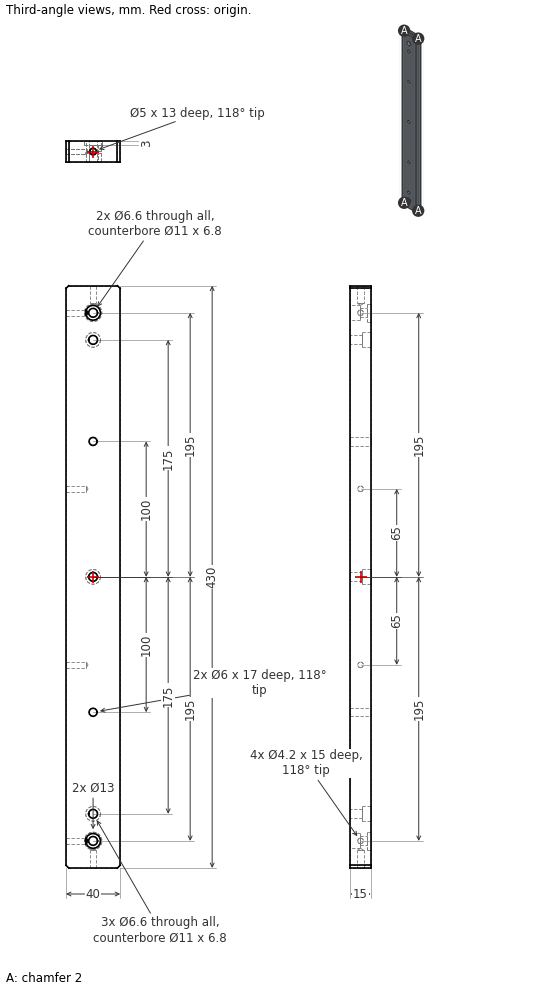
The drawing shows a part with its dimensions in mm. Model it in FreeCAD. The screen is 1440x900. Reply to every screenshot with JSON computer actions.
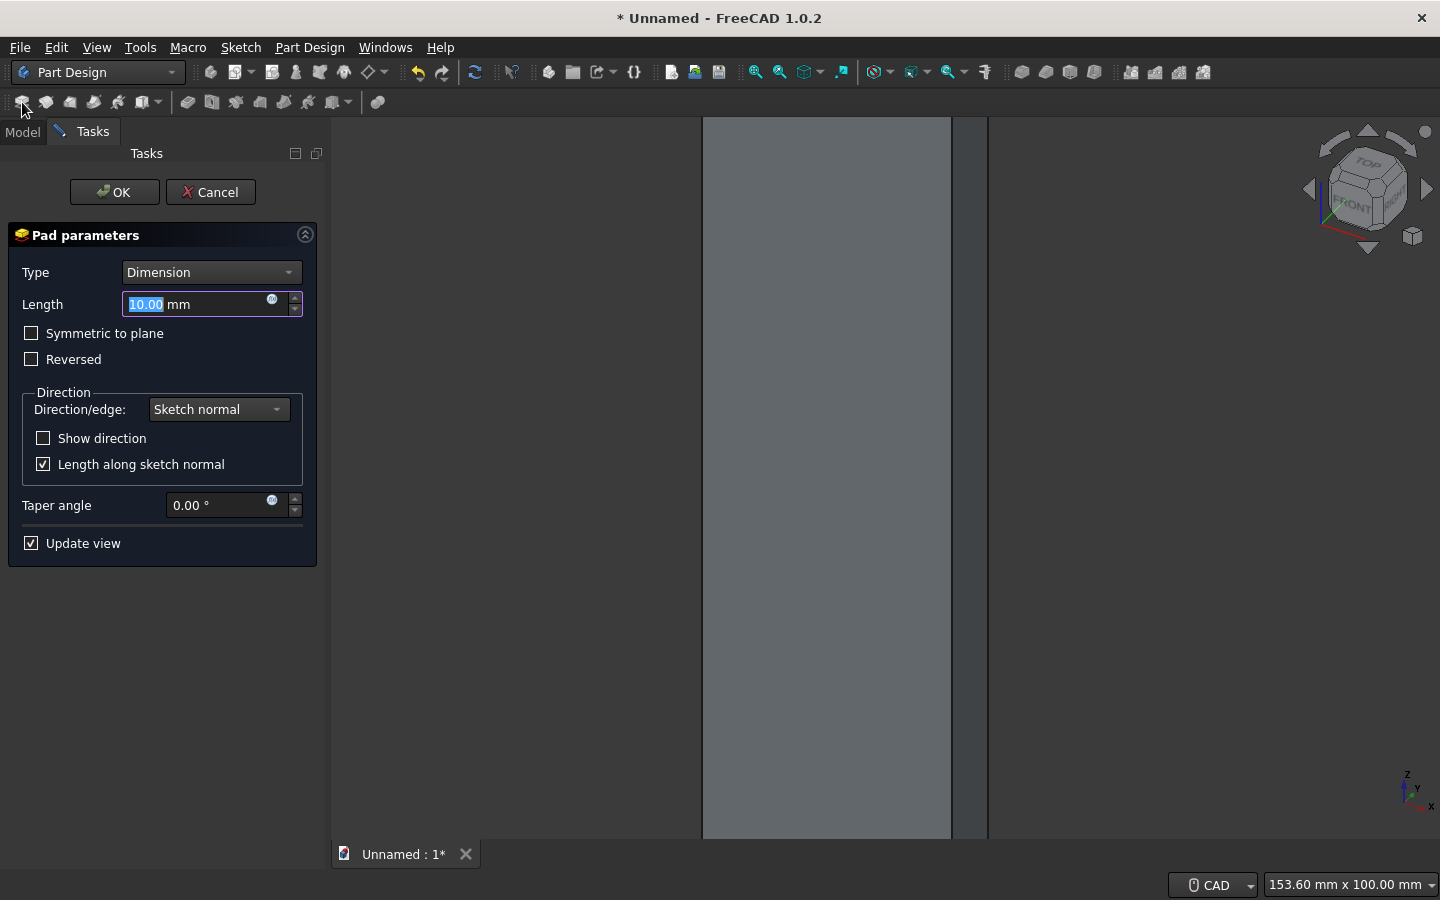
{"action": "type", "text": "15"}
{"action": "key", "text": "Tab"}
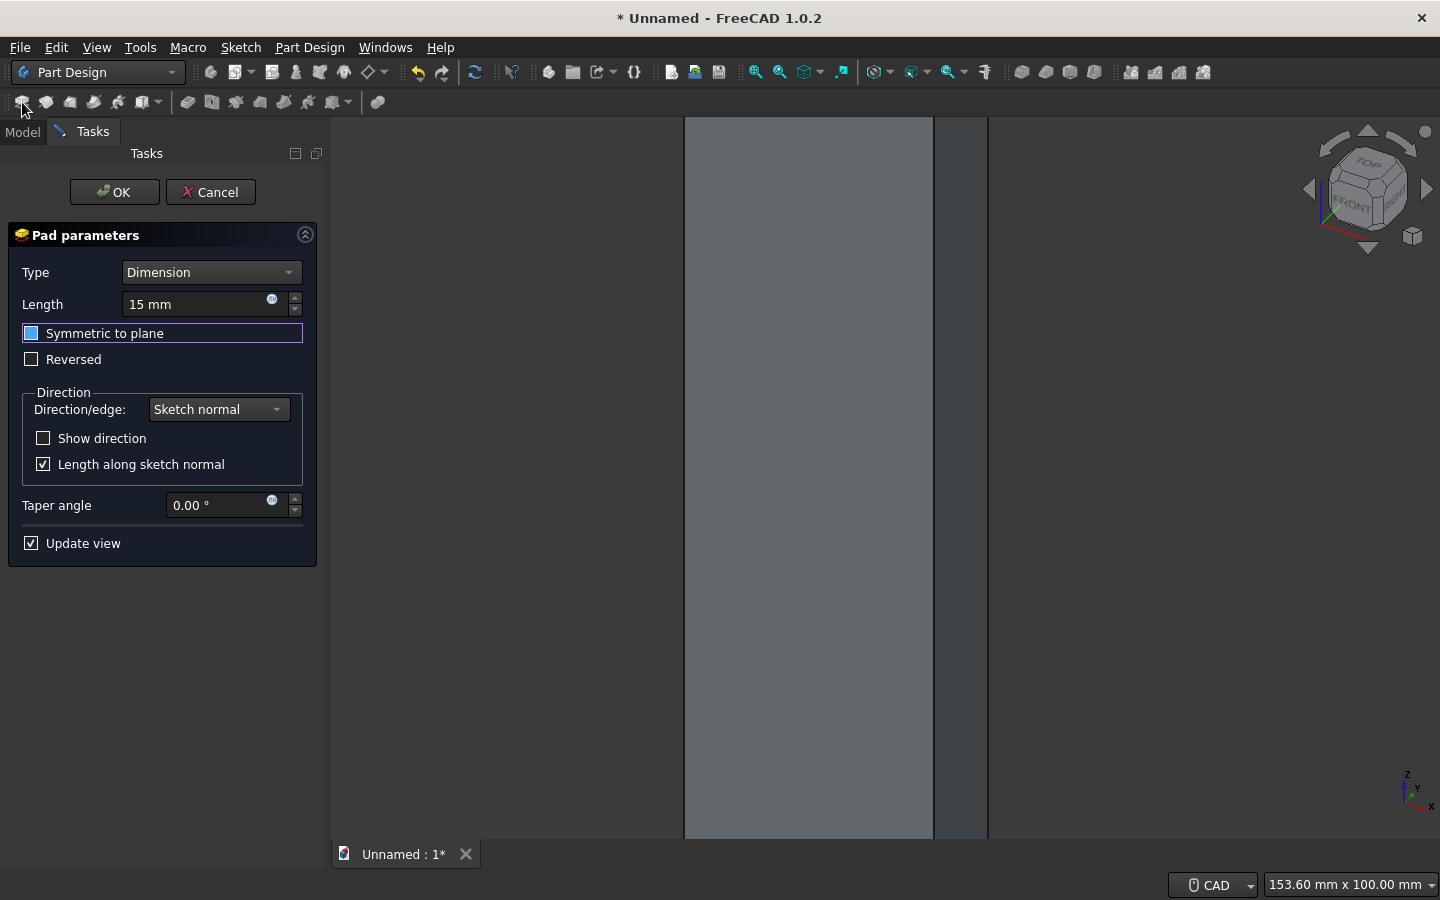
{"action": "left_click", "coordinate": [30, 333]}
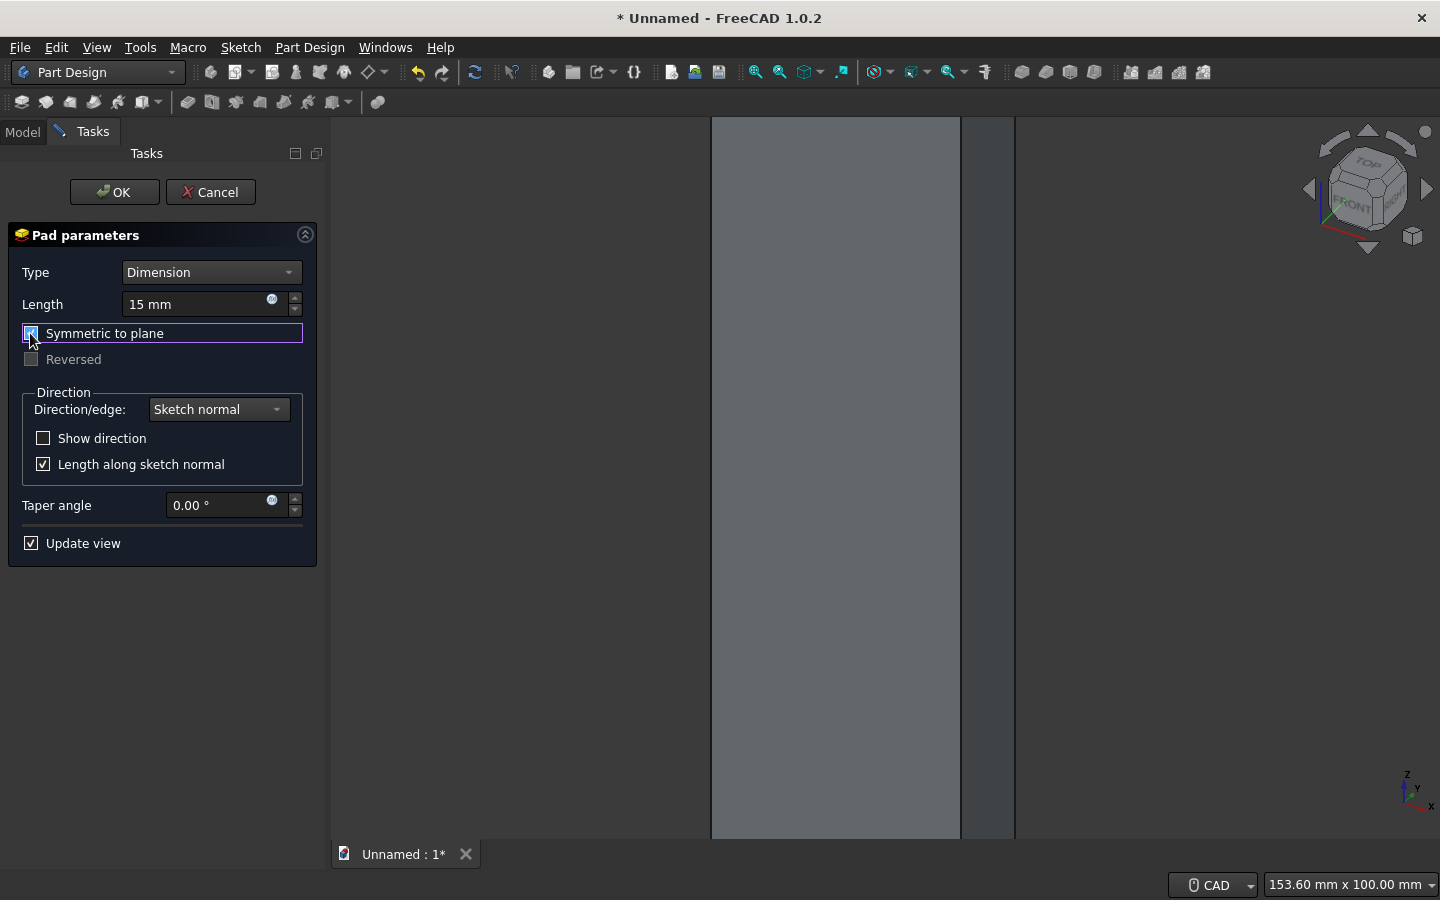
{"action": "left_click", "coordinate": [115, 192]}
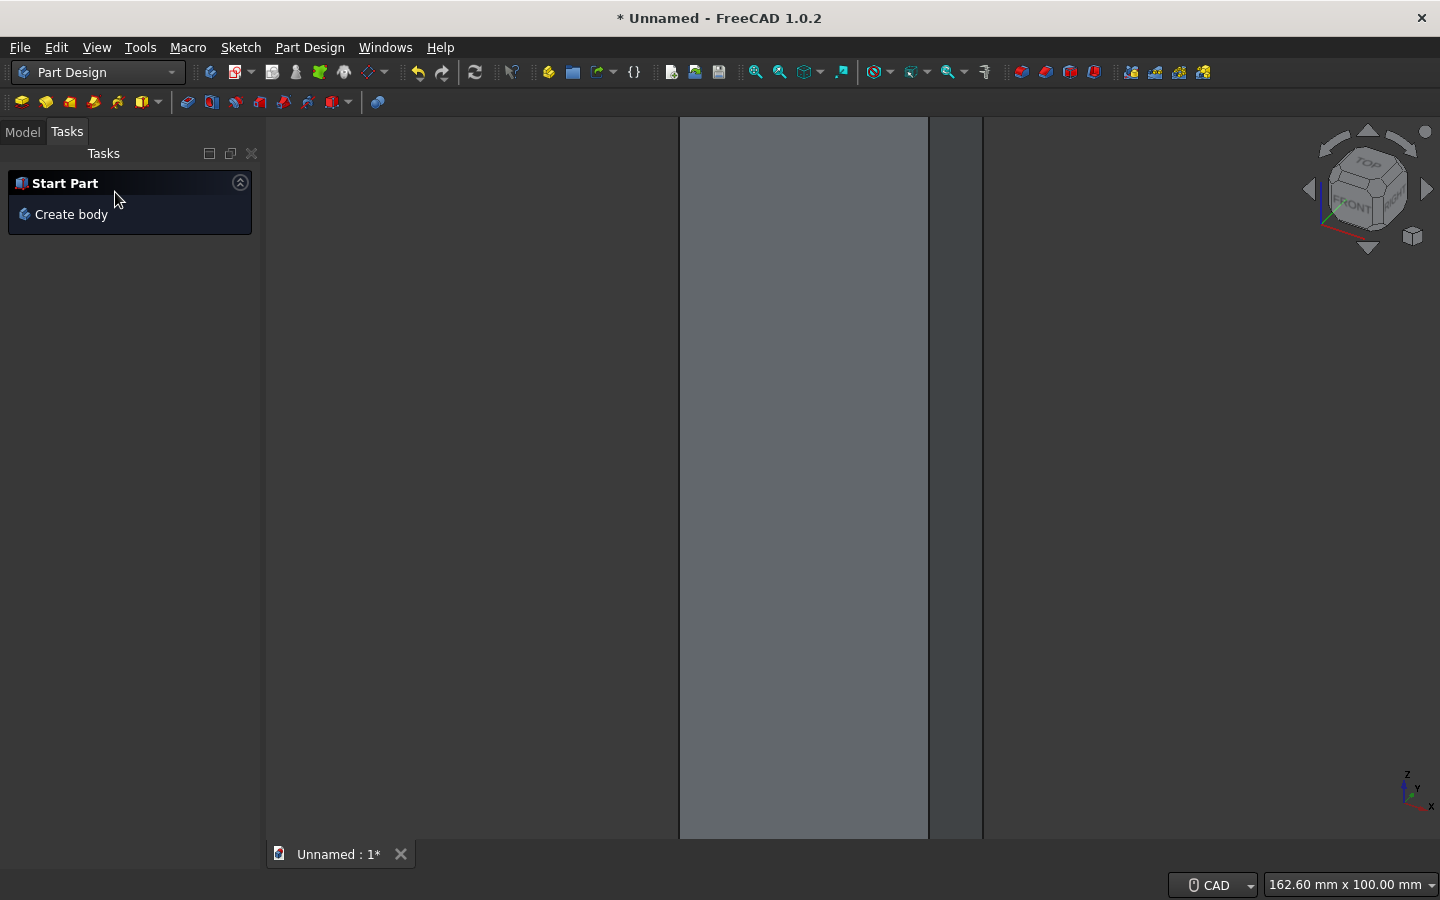
{"action": "key", "text": "v f"}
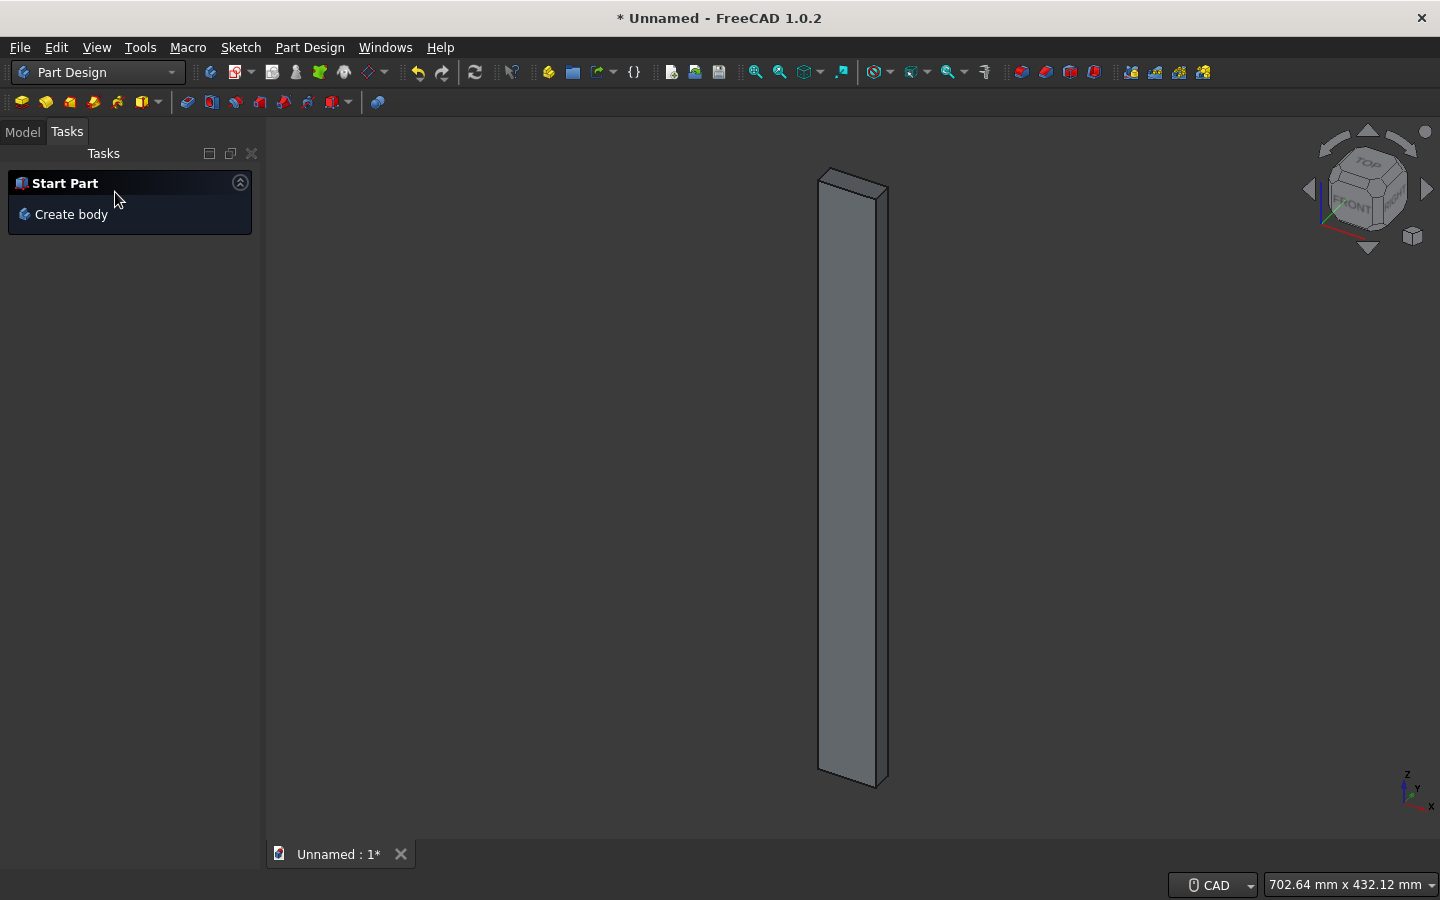
{"action": "key", "text": "4"}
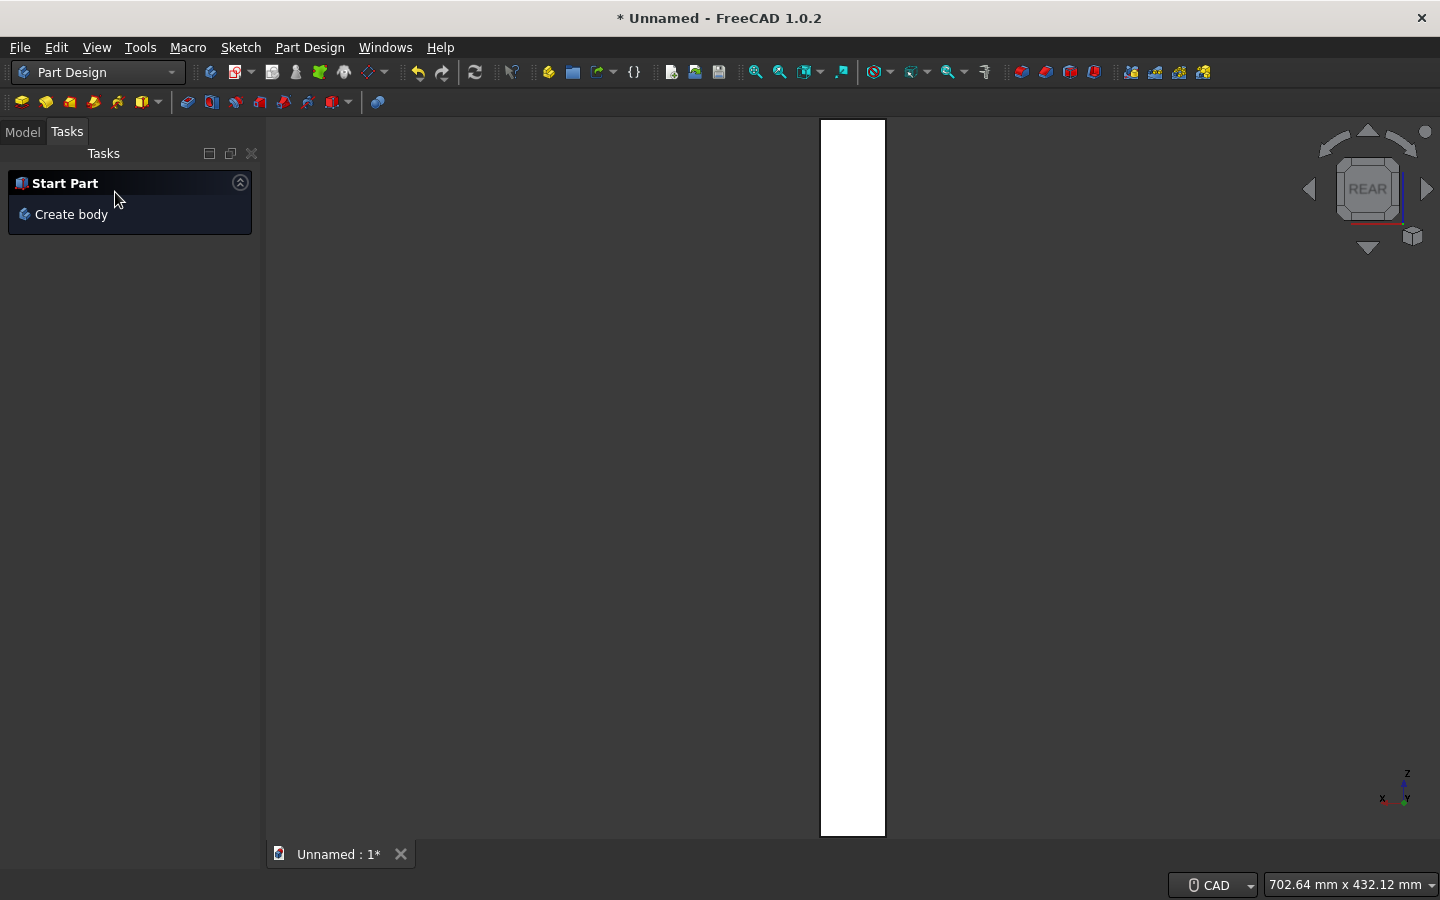
{"action": "left_click", "coordinate": [853, 169]}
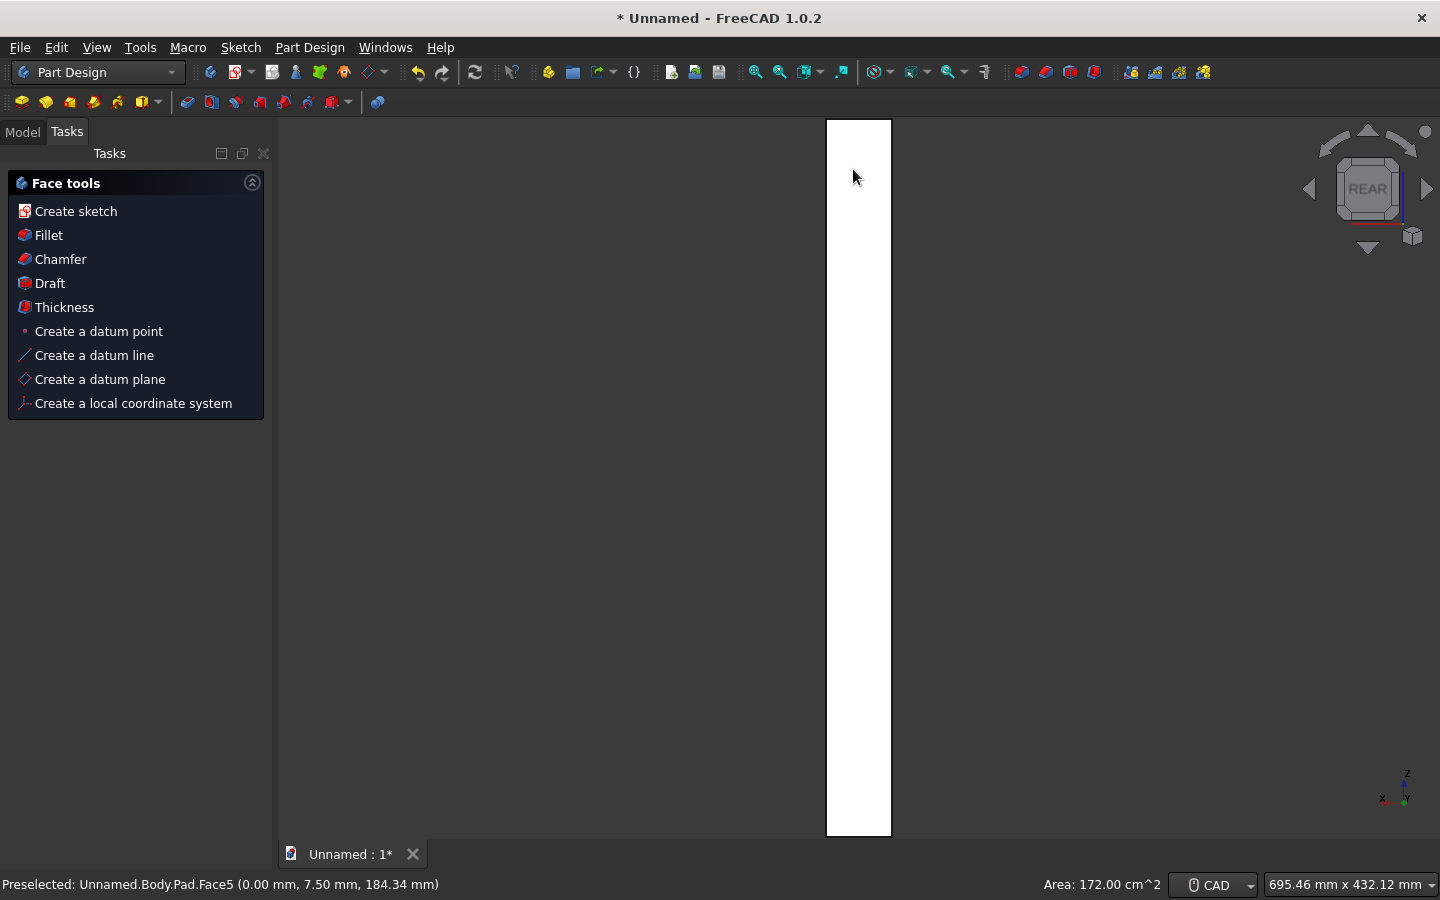
{"action": "left_click", "coordinate": [236, 72]}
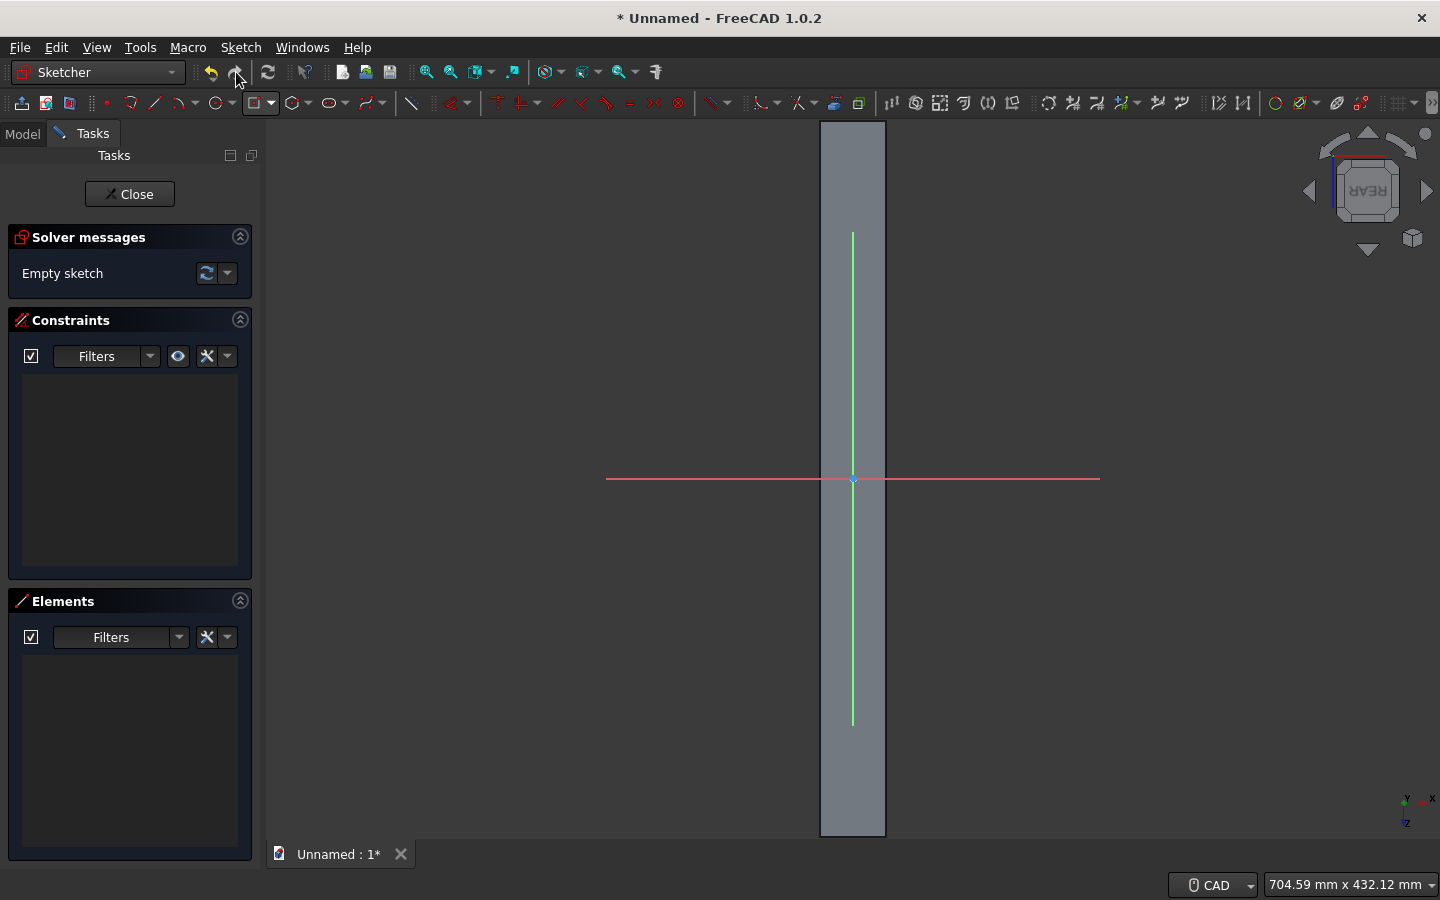
{"action": "scroll", "coordinate": [645, 479], "scroll_direction": "down", "scroll_amount": 2}